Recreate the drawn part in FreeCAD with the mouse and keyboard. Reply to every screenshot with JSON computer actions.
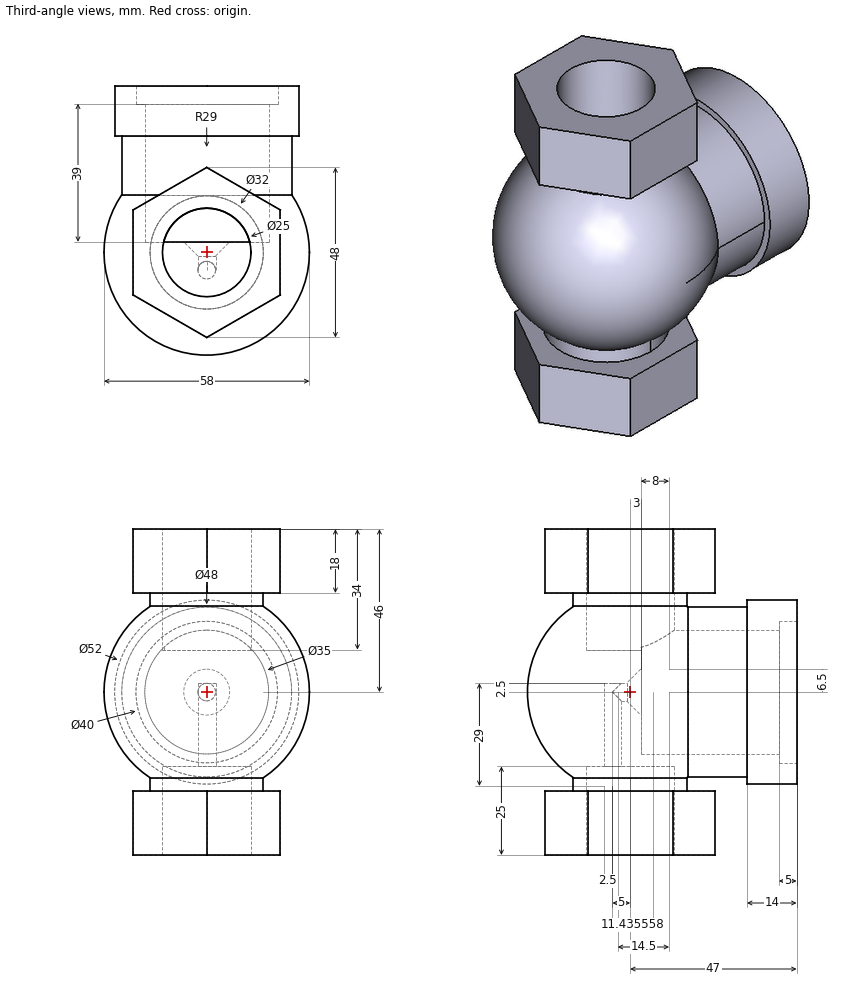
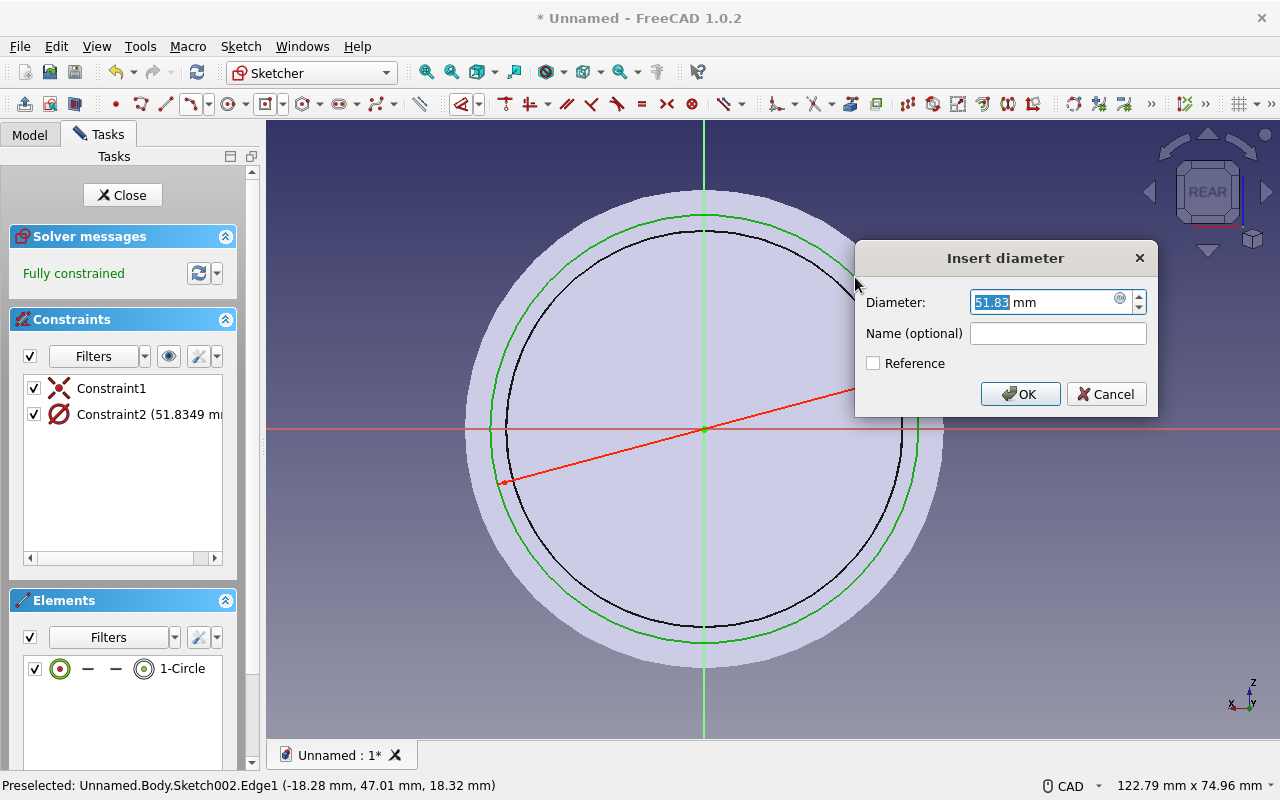
{"action": "type", "text": "52"}
{"action": "key", "text": "Return"}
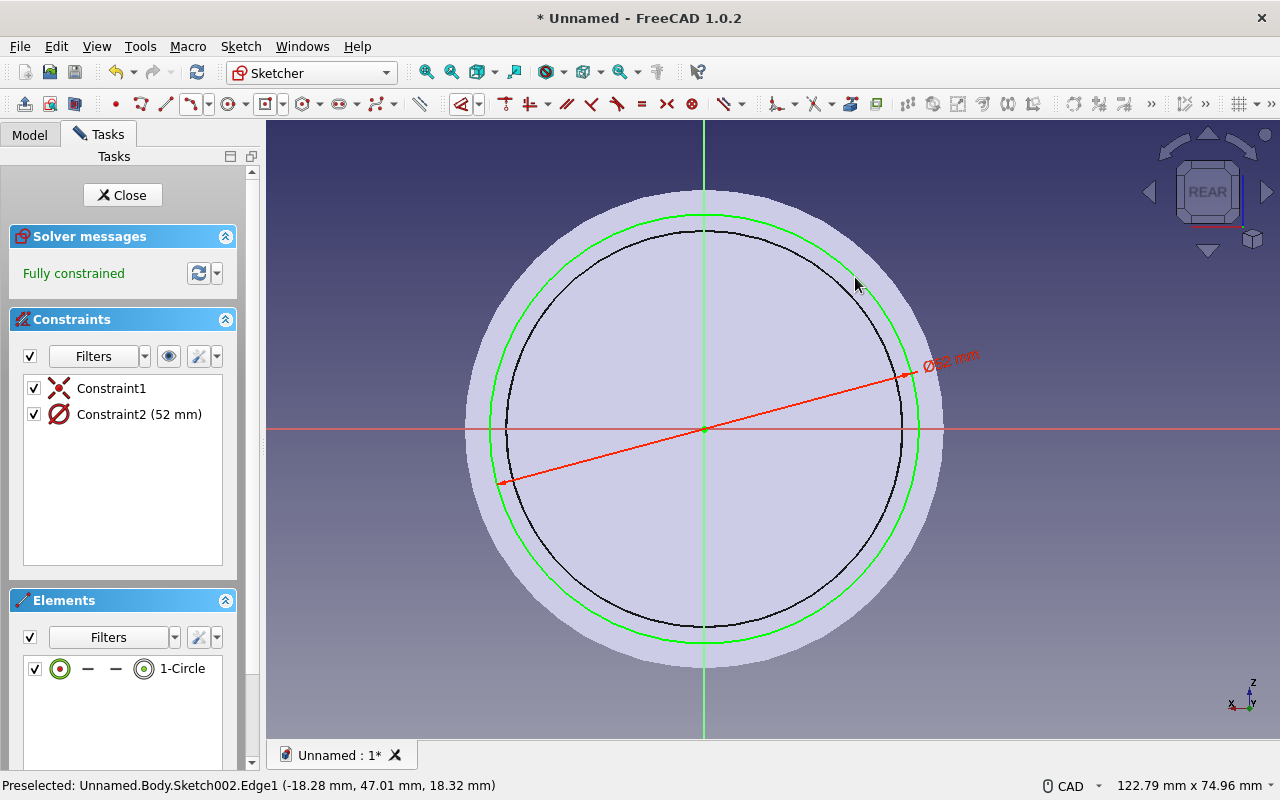
{"action": "left_click", "coordinate": [123, 195]}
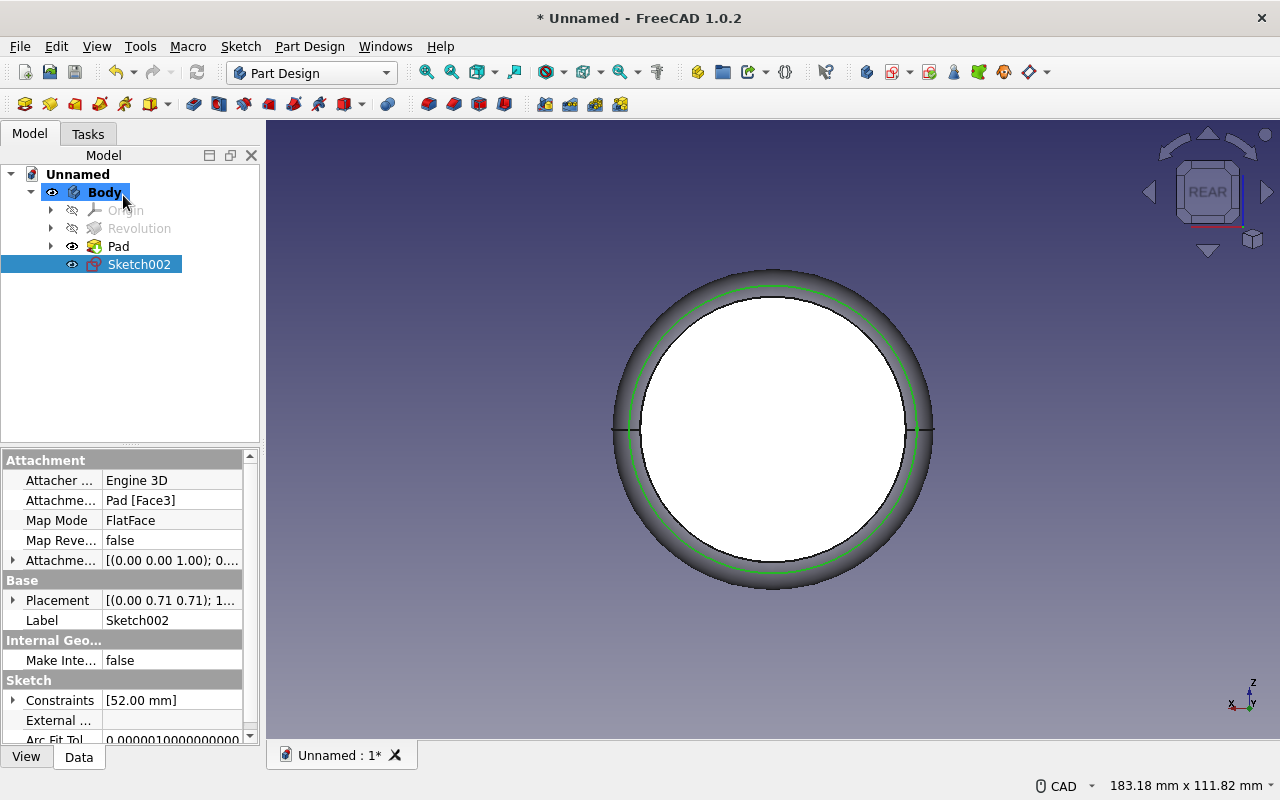
{"action": "left_click", "coordinate": [25, 104]}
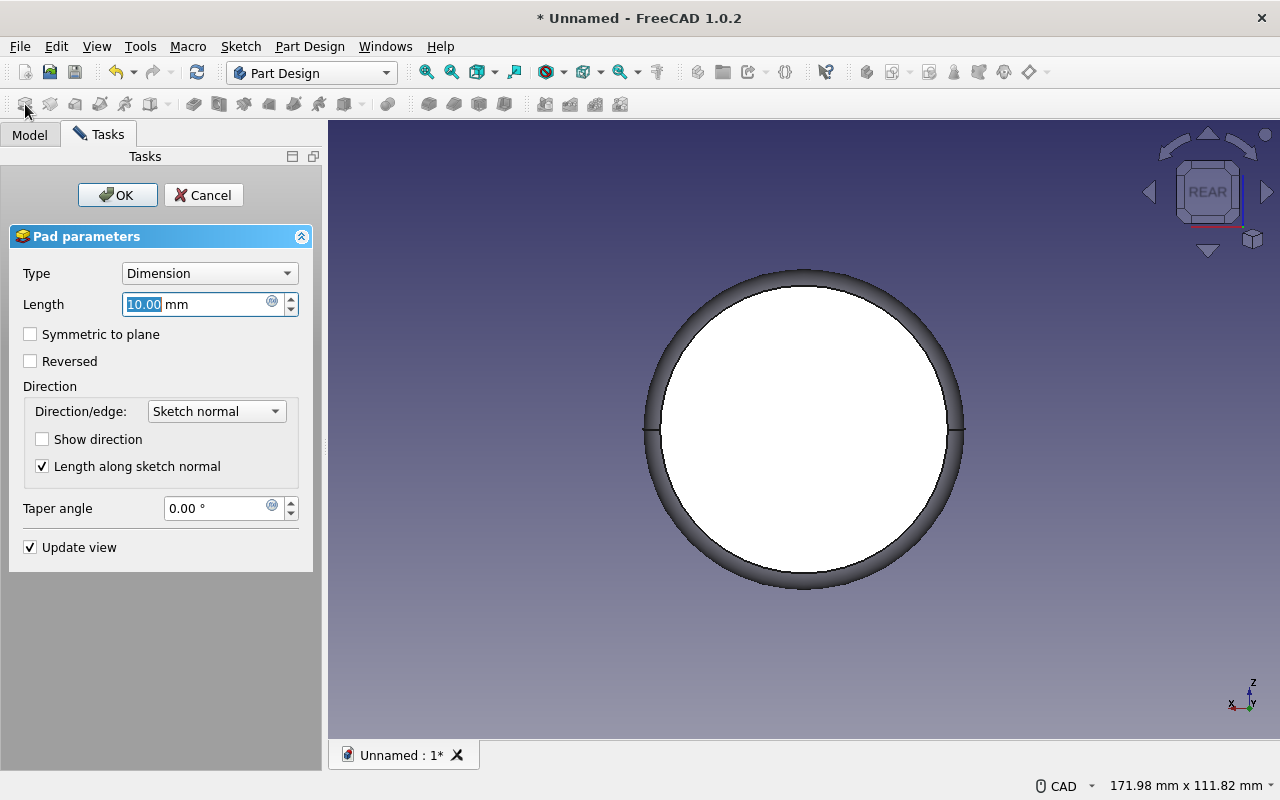
{"action": "type", "text": "14"}
{"action": "key", "text": "Tab"}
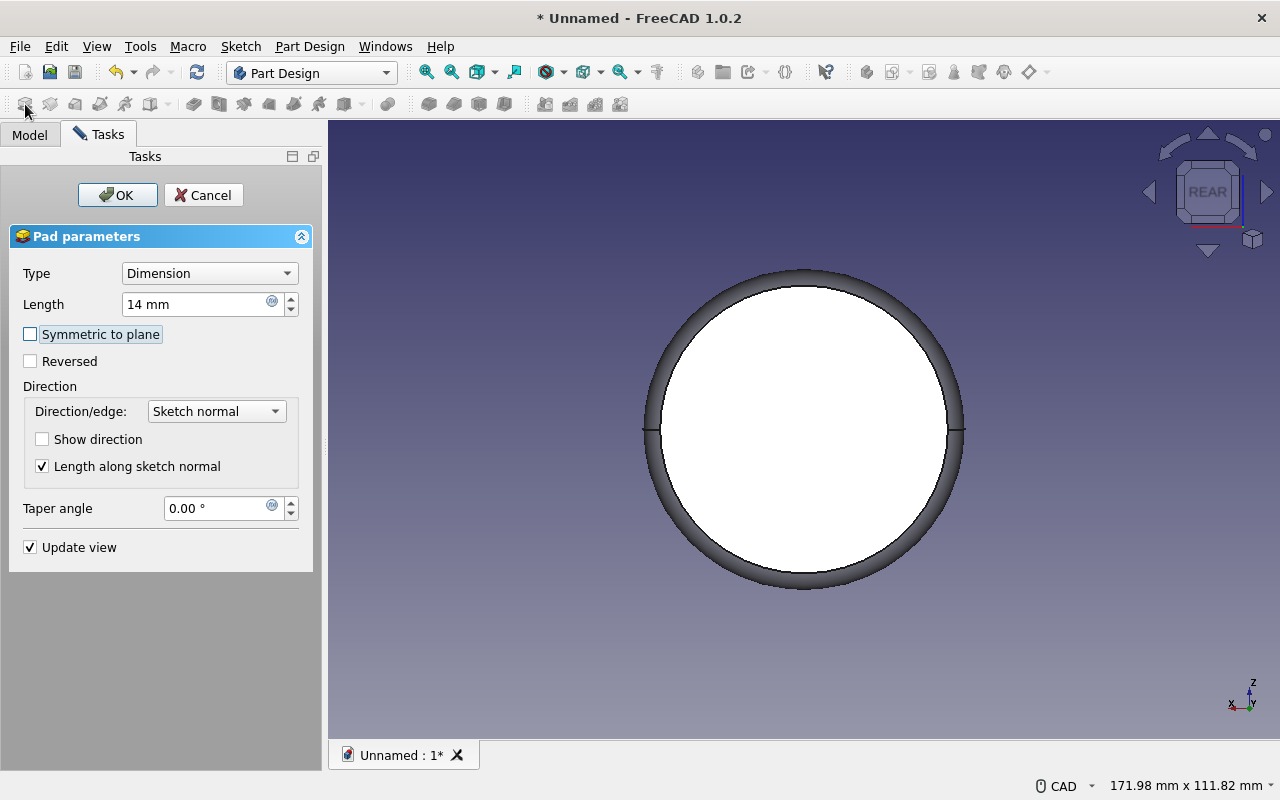
{"action": "left_click", "coordinate": [31, 361]}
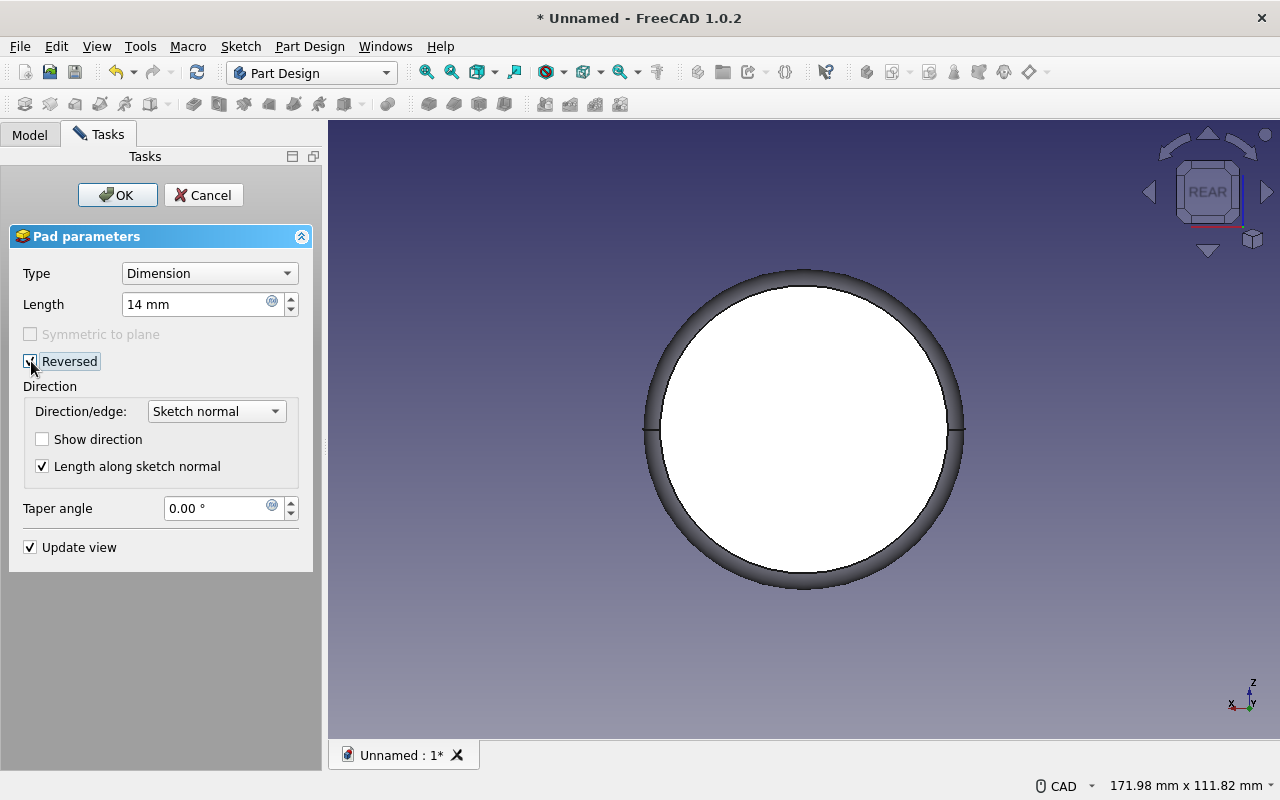
{"action": "left_click", "coordinate": [118, 195]}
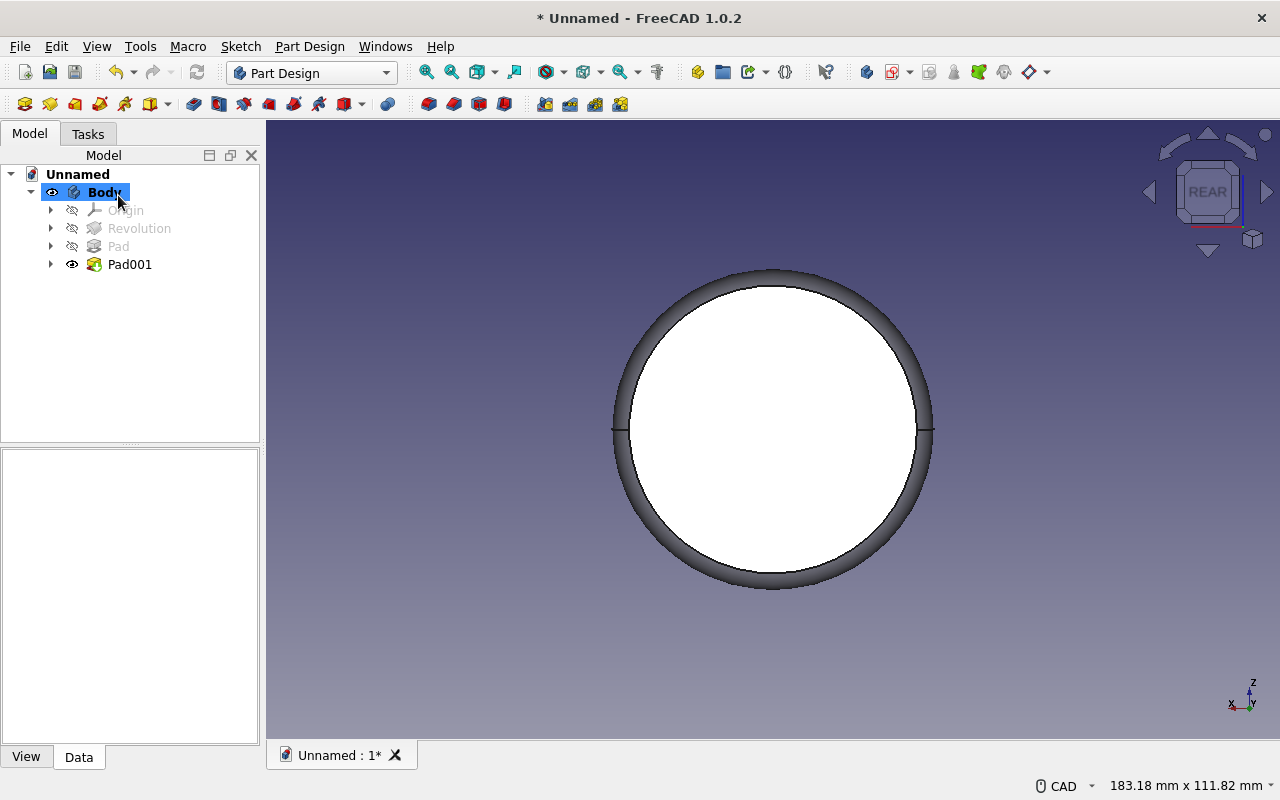
{"action": "left_click", "coordinate": [892, 72]}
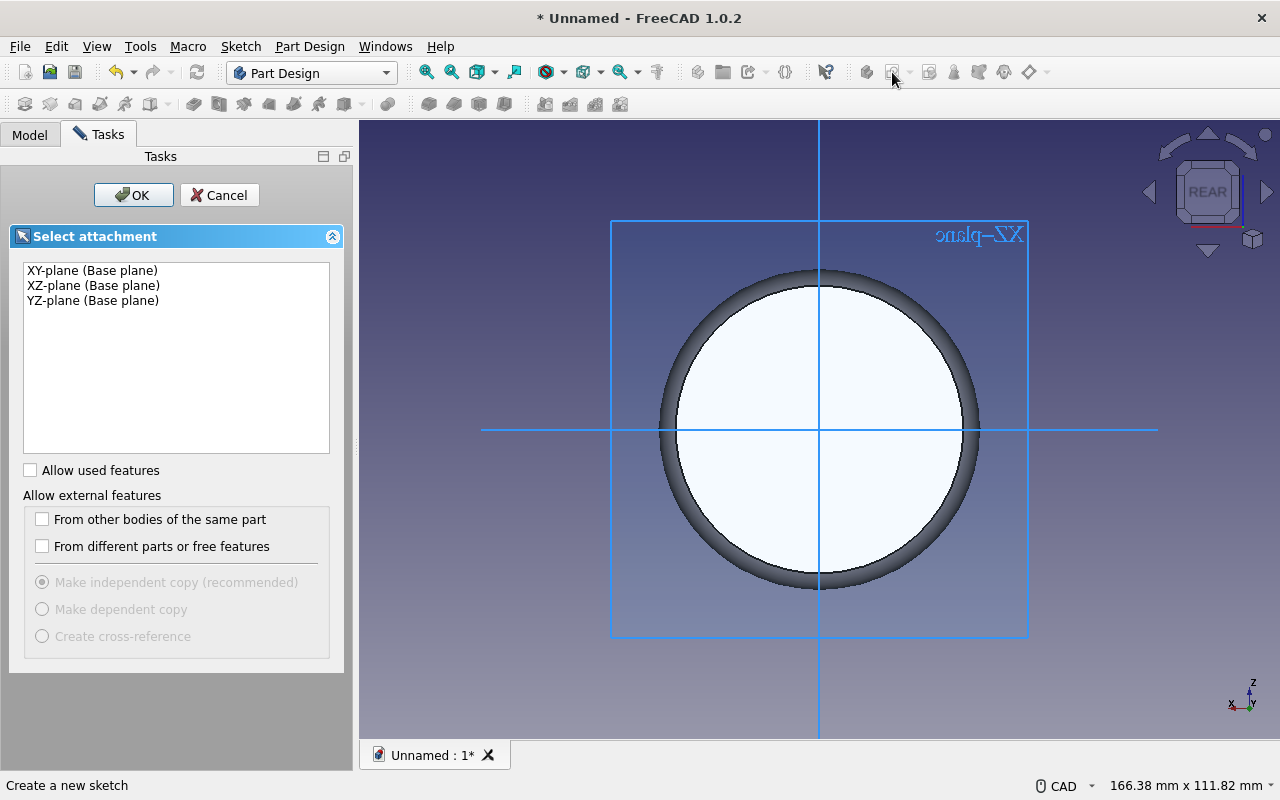
{"action": "left_click", "coordinate": [84, 270]}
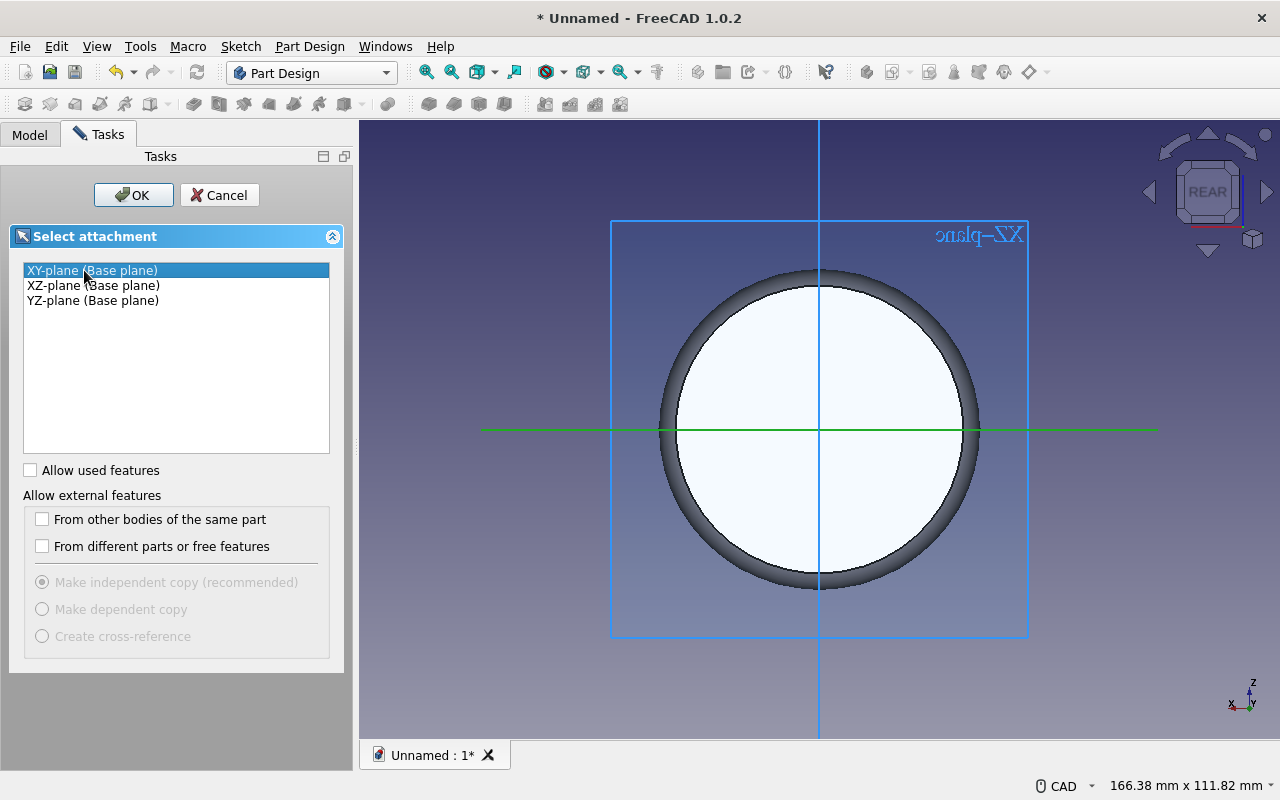
{"action": "left_click", "coordinate": [134, 195]}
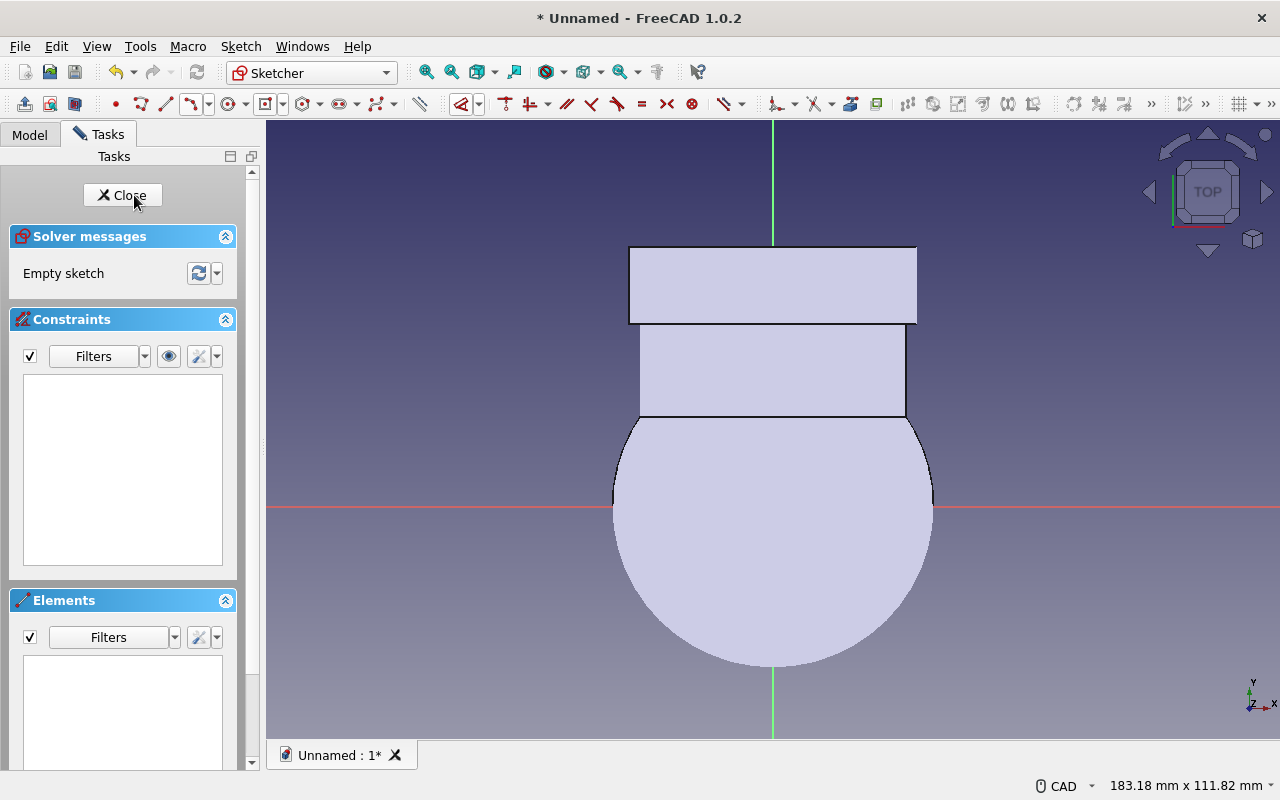
{"action": "key", "text": "q s"}